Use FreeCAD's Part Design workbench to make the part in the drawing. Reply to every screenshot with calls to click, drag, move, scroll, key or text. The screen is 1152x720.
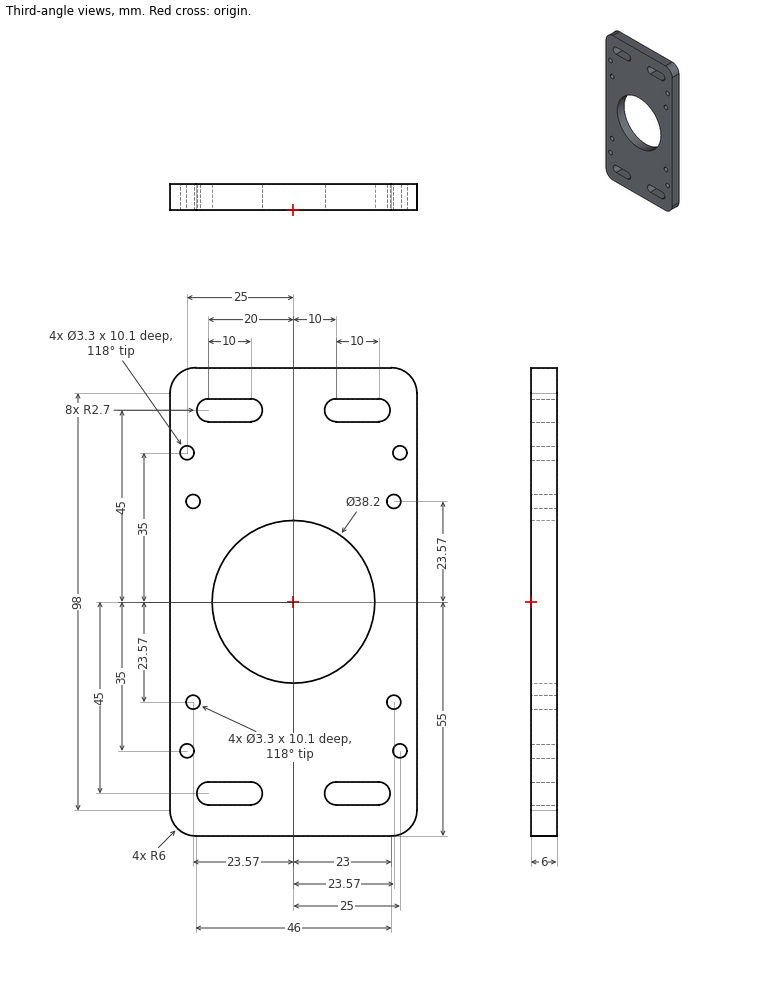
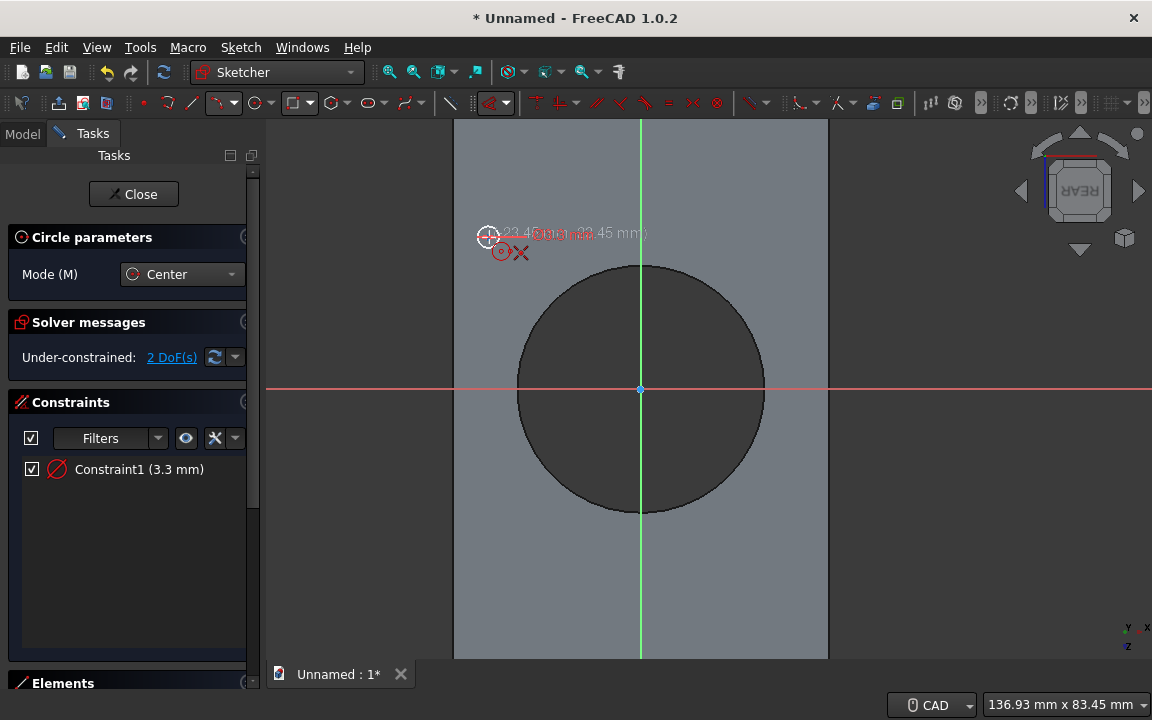
scroll(793, 237, up, 4)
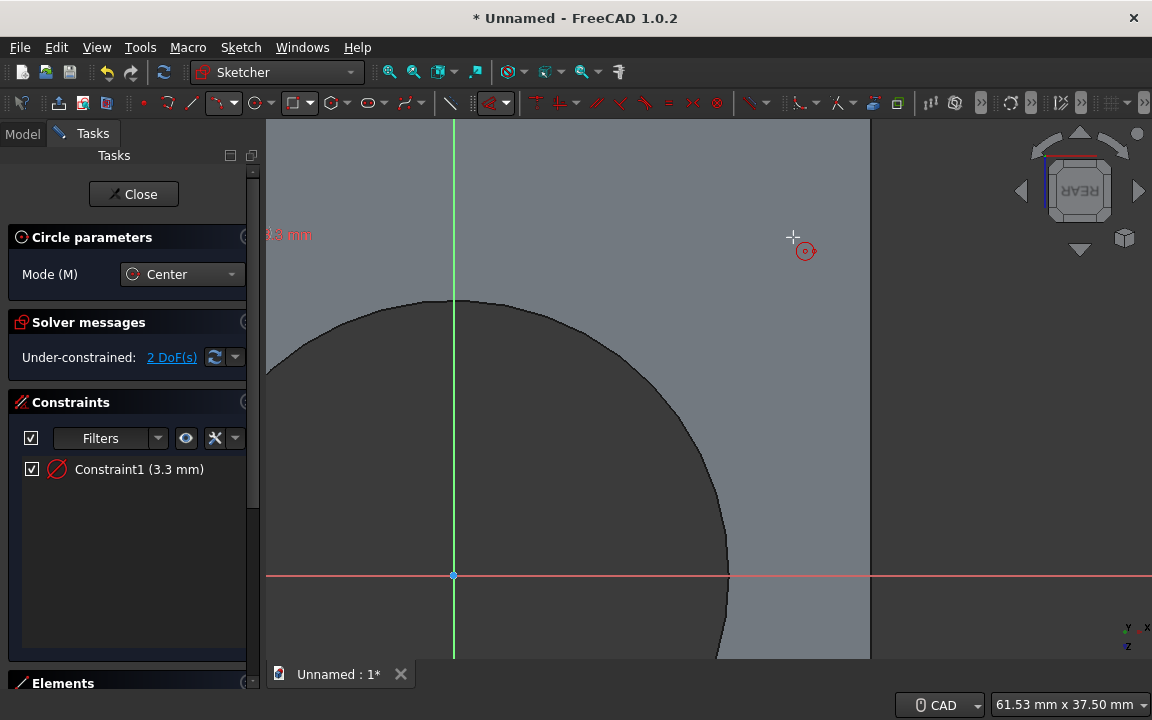
click(793, 236)
move(810, 219)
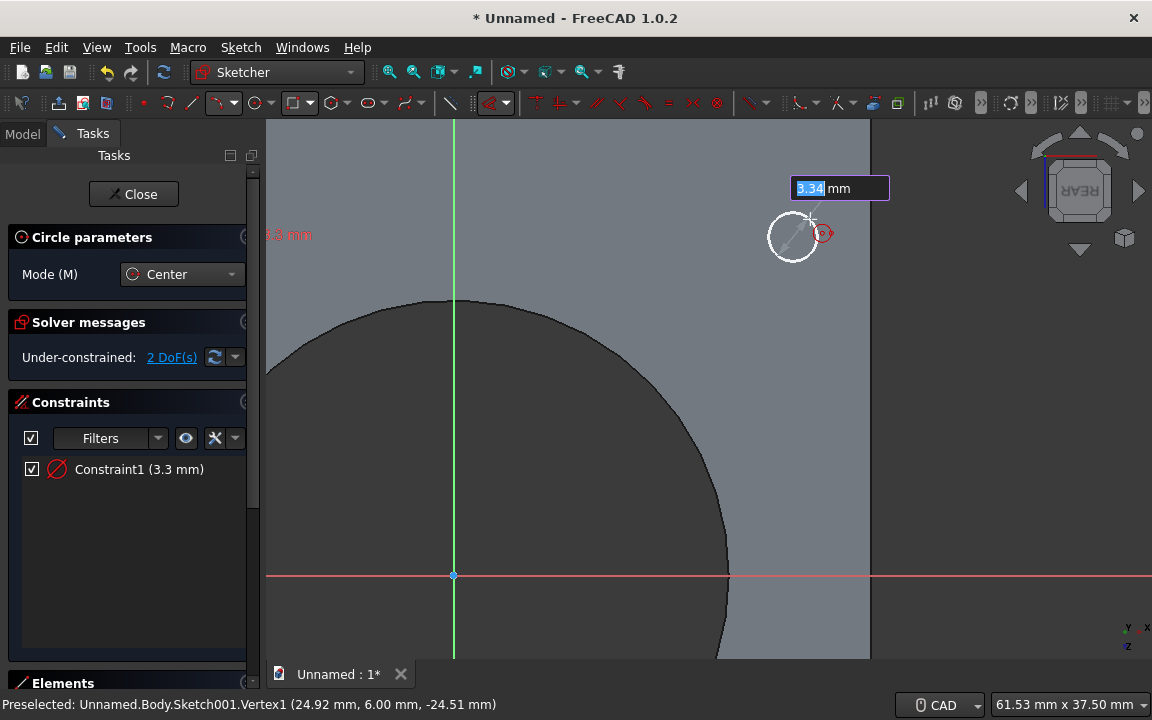
text(3.3)
key(Return)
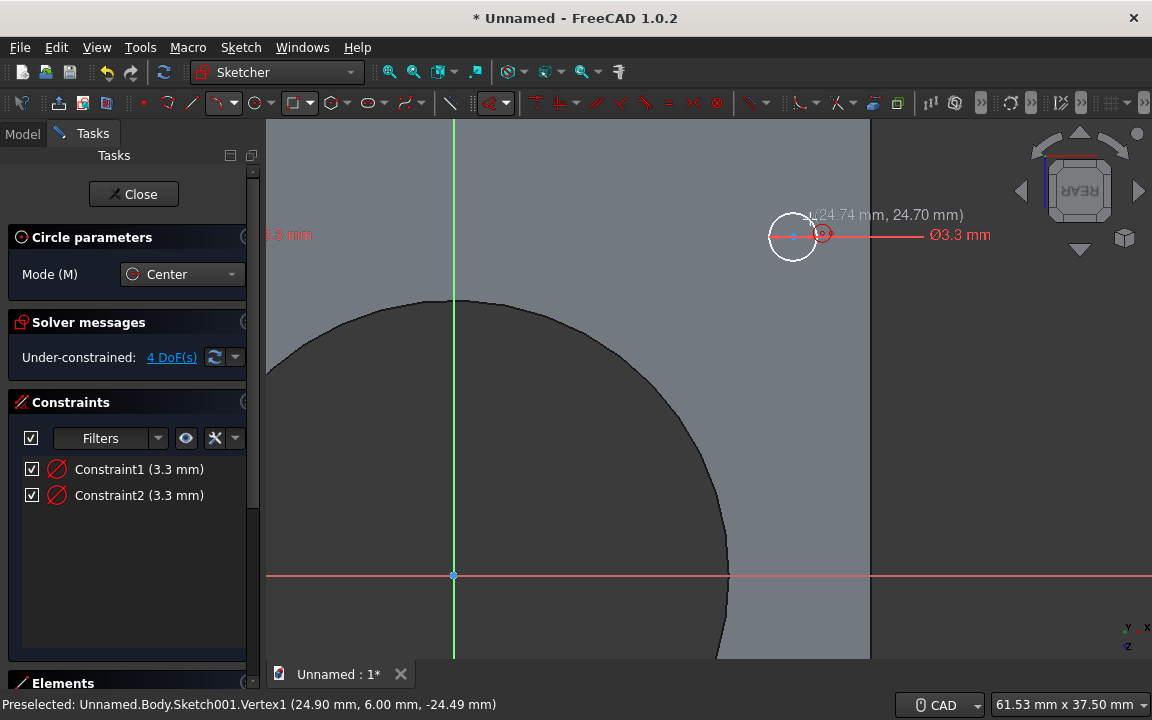
scroll(793, 237, down, 4)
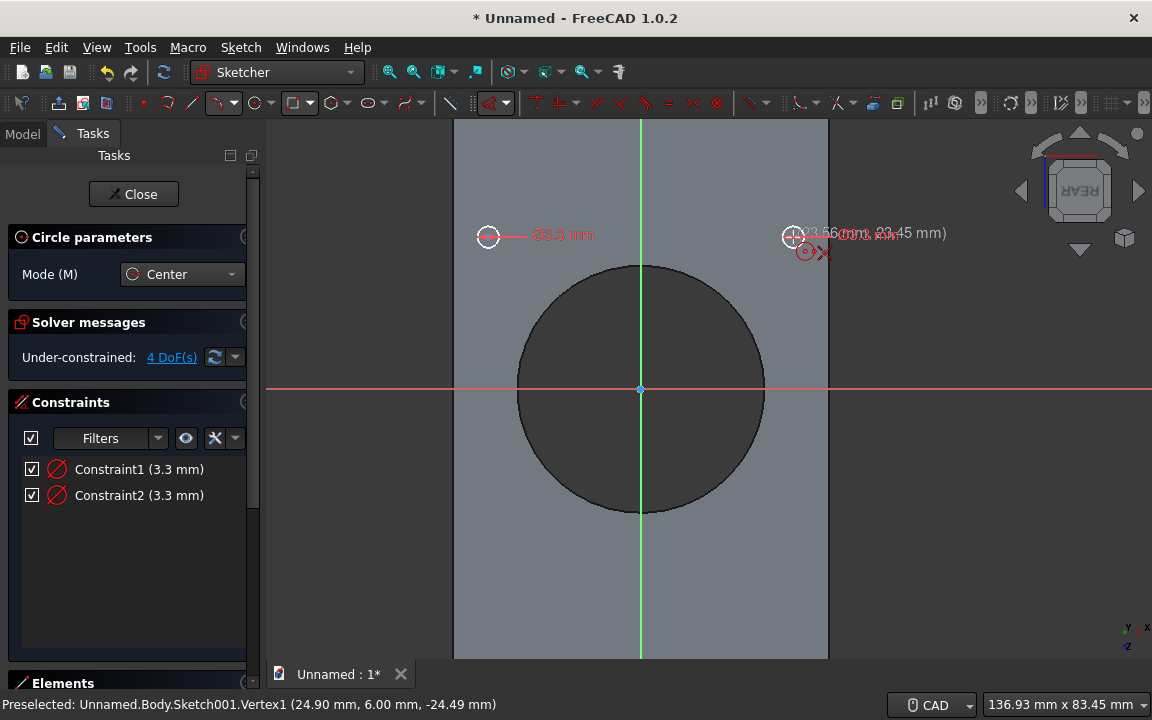
scroll(793, 542, up, 4)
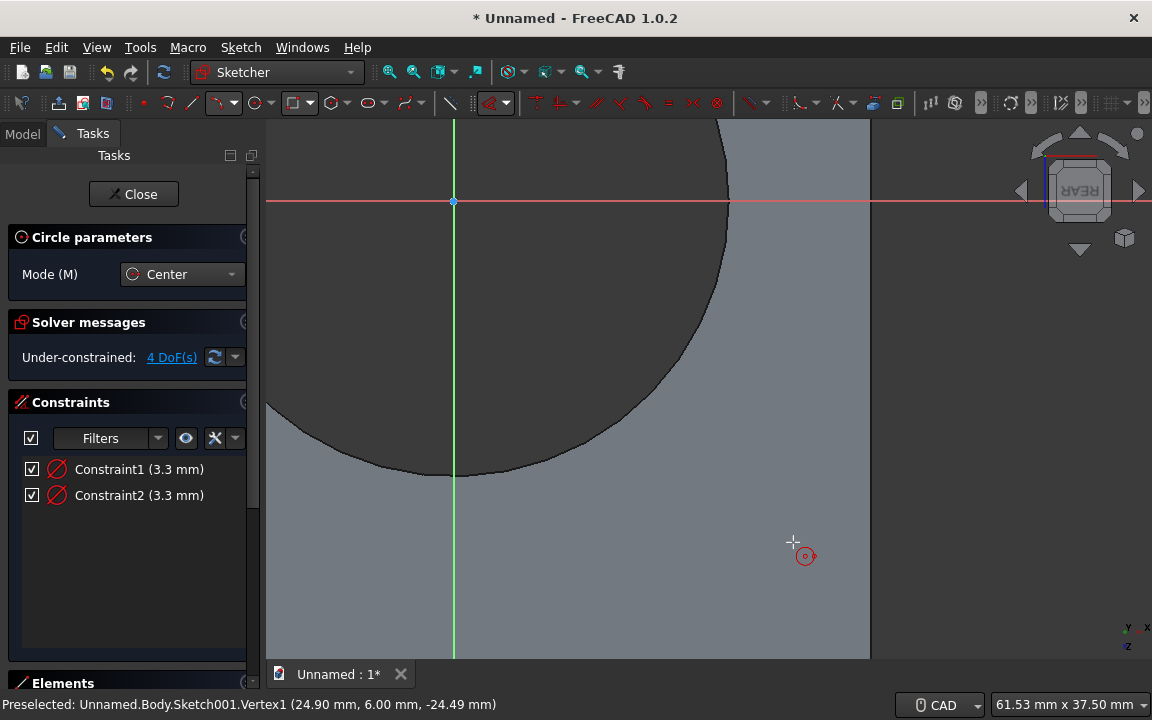
click(793, 541)
move(810, 524)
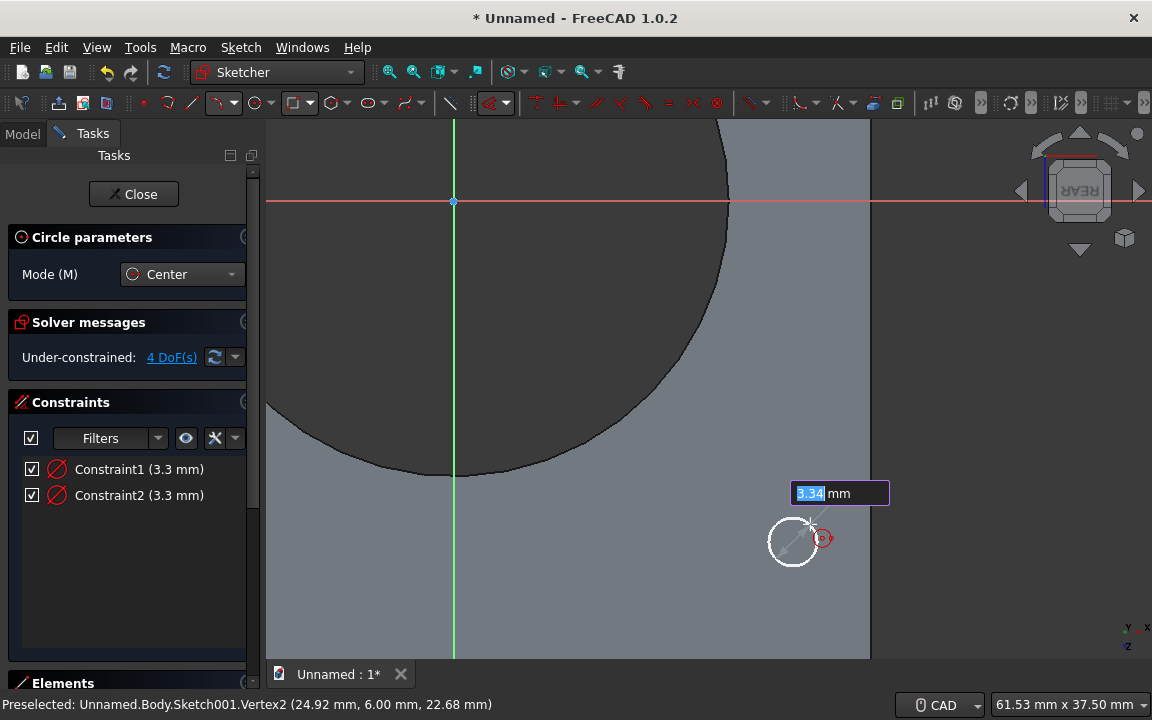
text(3.3)
key(Return)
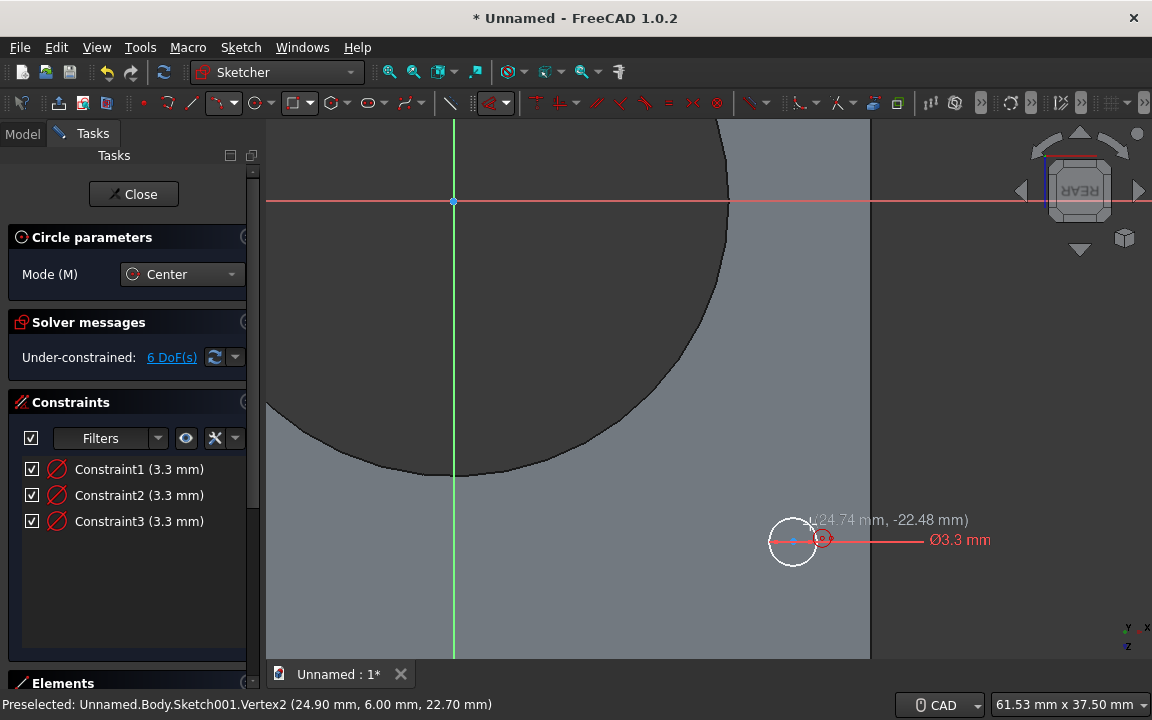
scroll(793, 542, down, 4)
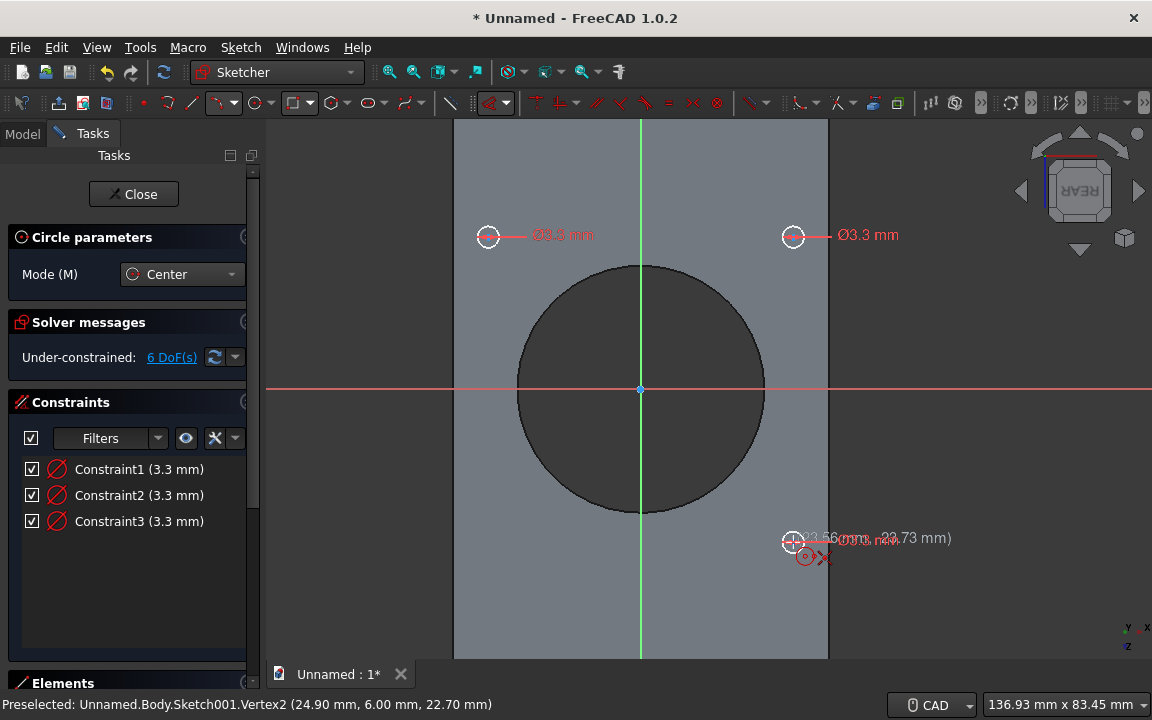
scroll(488, 542, up, 4)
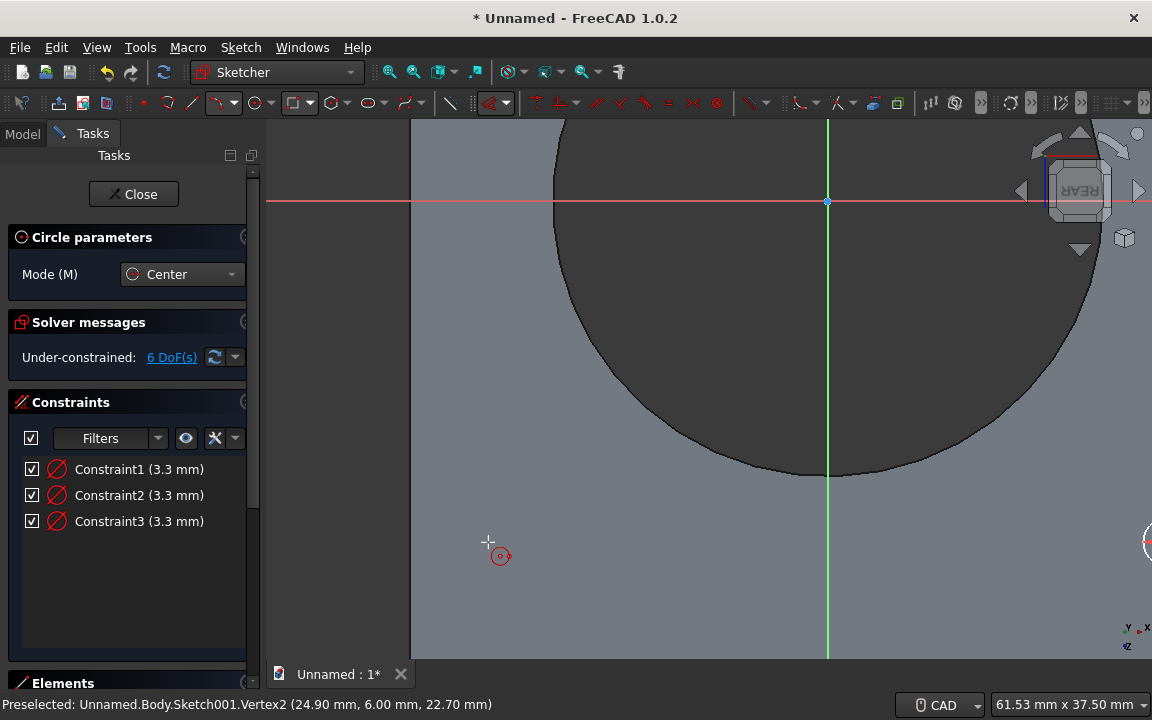
click(488, 541)
move(505, 524)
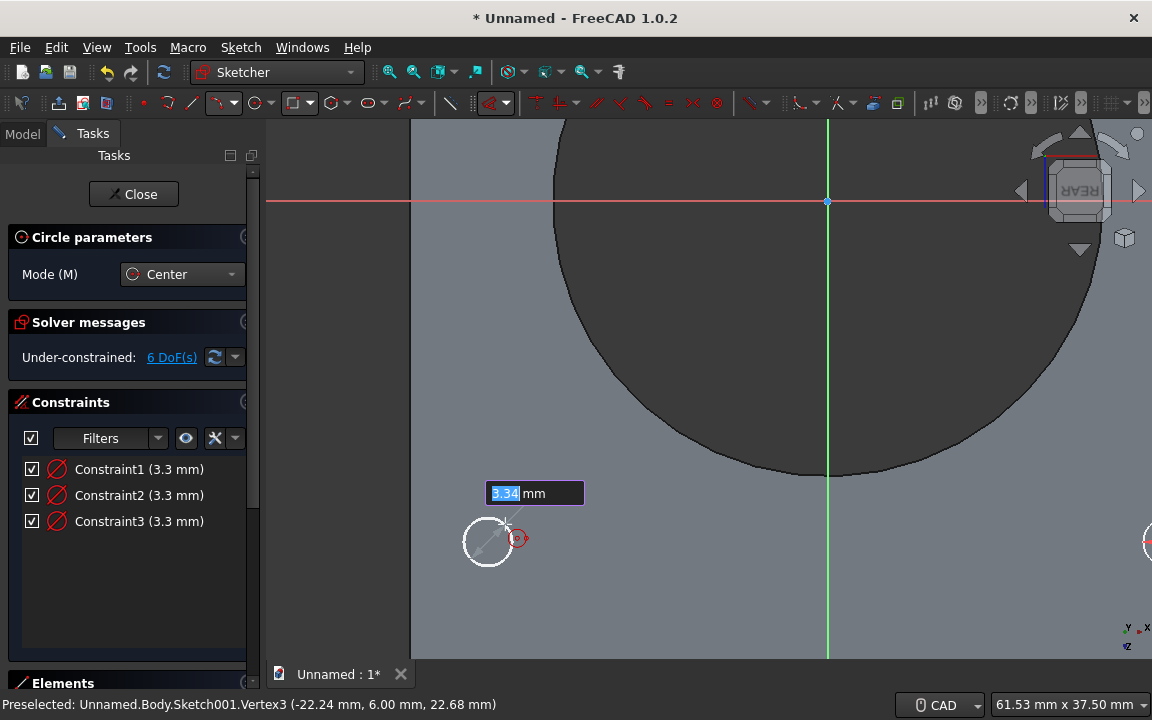
text(3.3)
key(Return)
key(Escape)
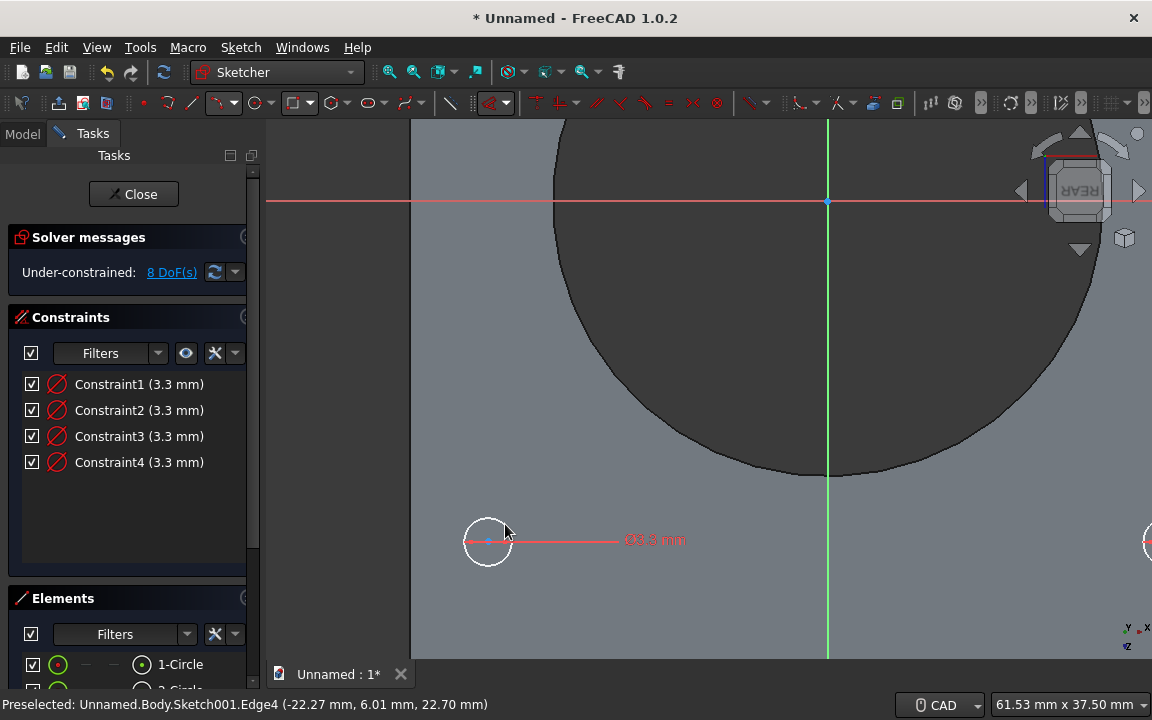
scroll(488, 542, down, 4)